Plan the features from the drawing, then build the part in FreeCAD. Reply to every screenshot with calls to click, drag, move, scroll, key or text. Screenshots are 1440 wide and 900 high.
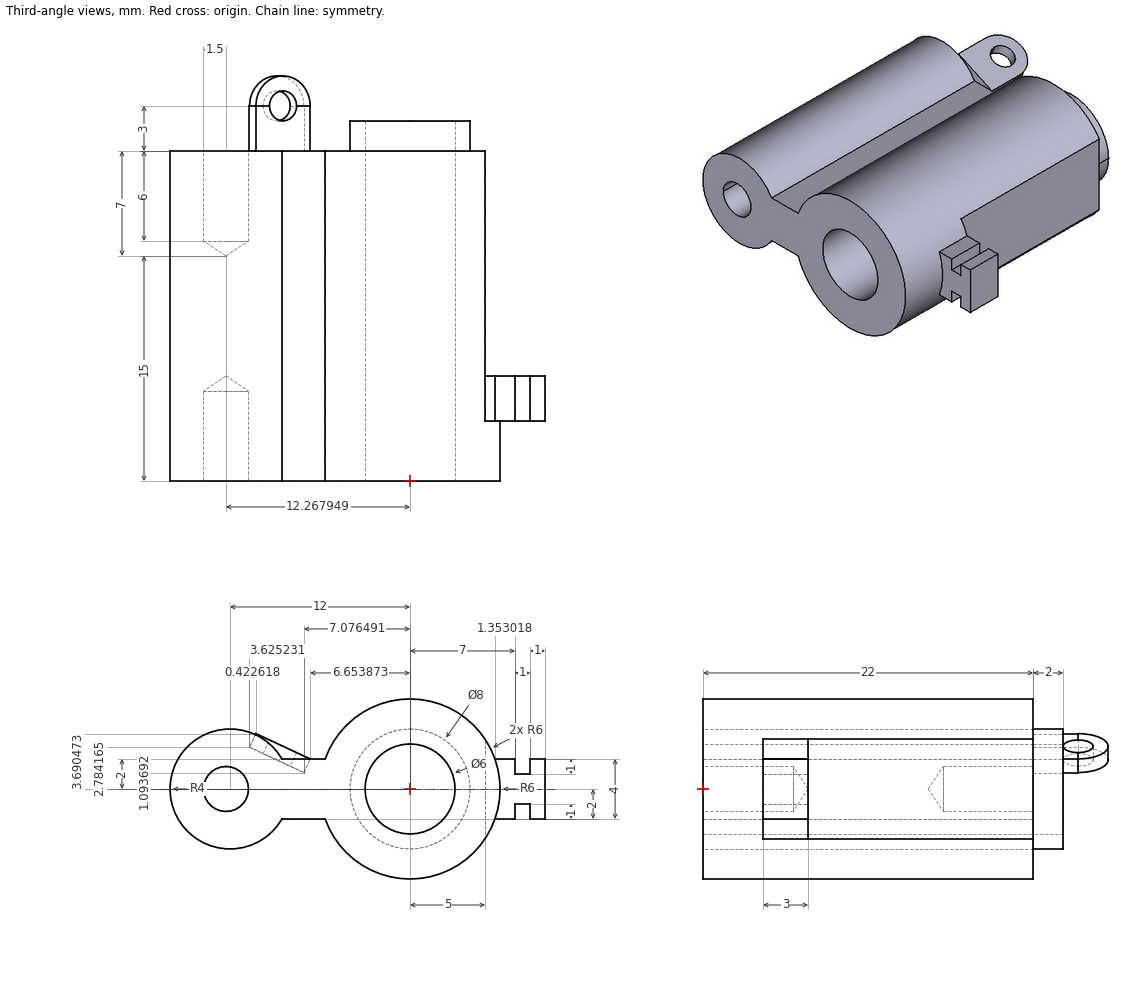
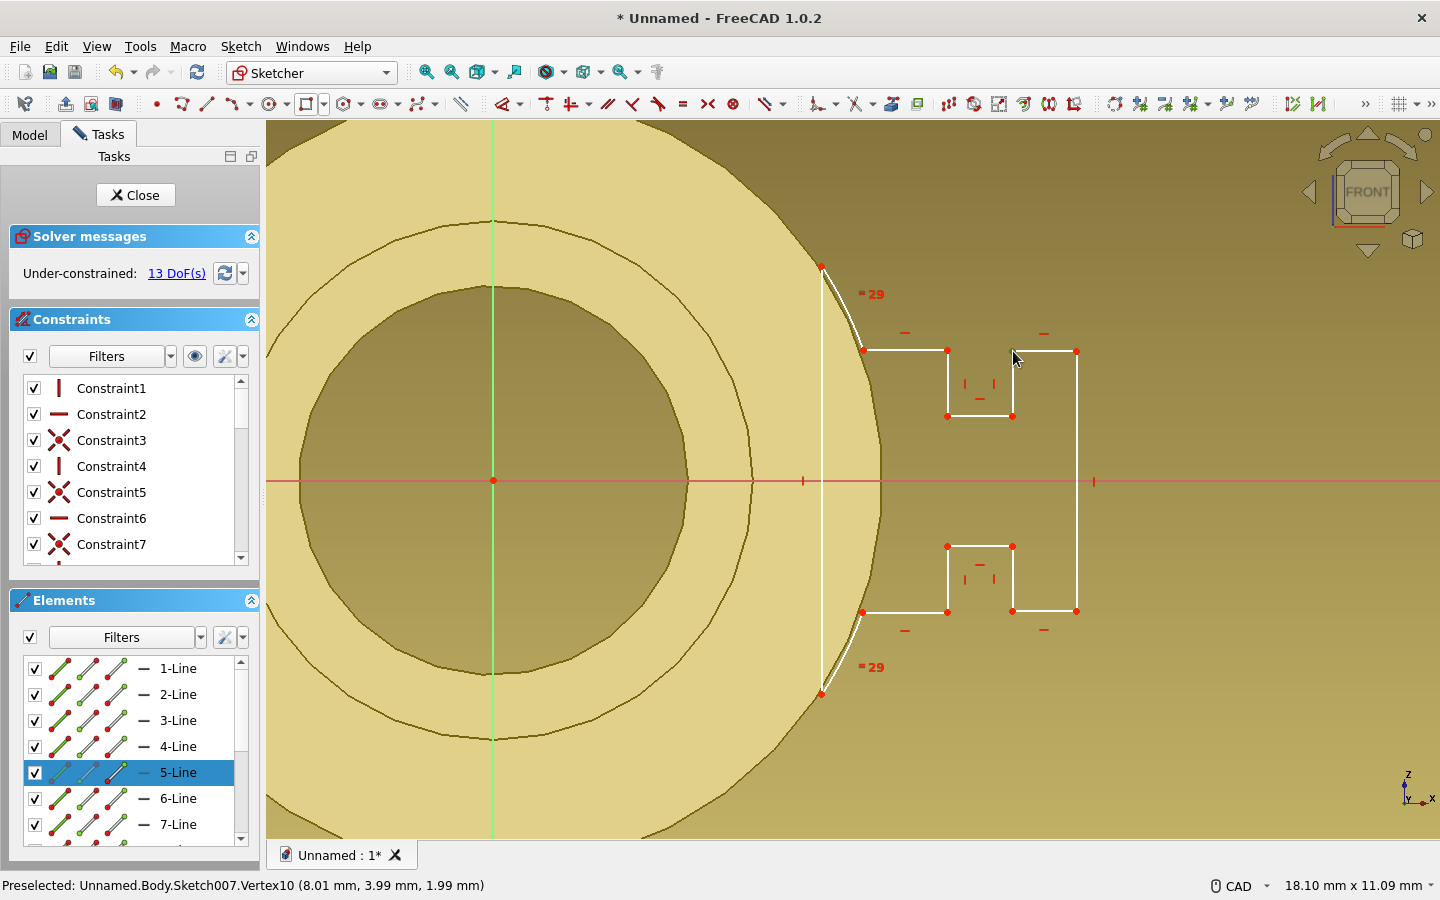
click(1013, 611)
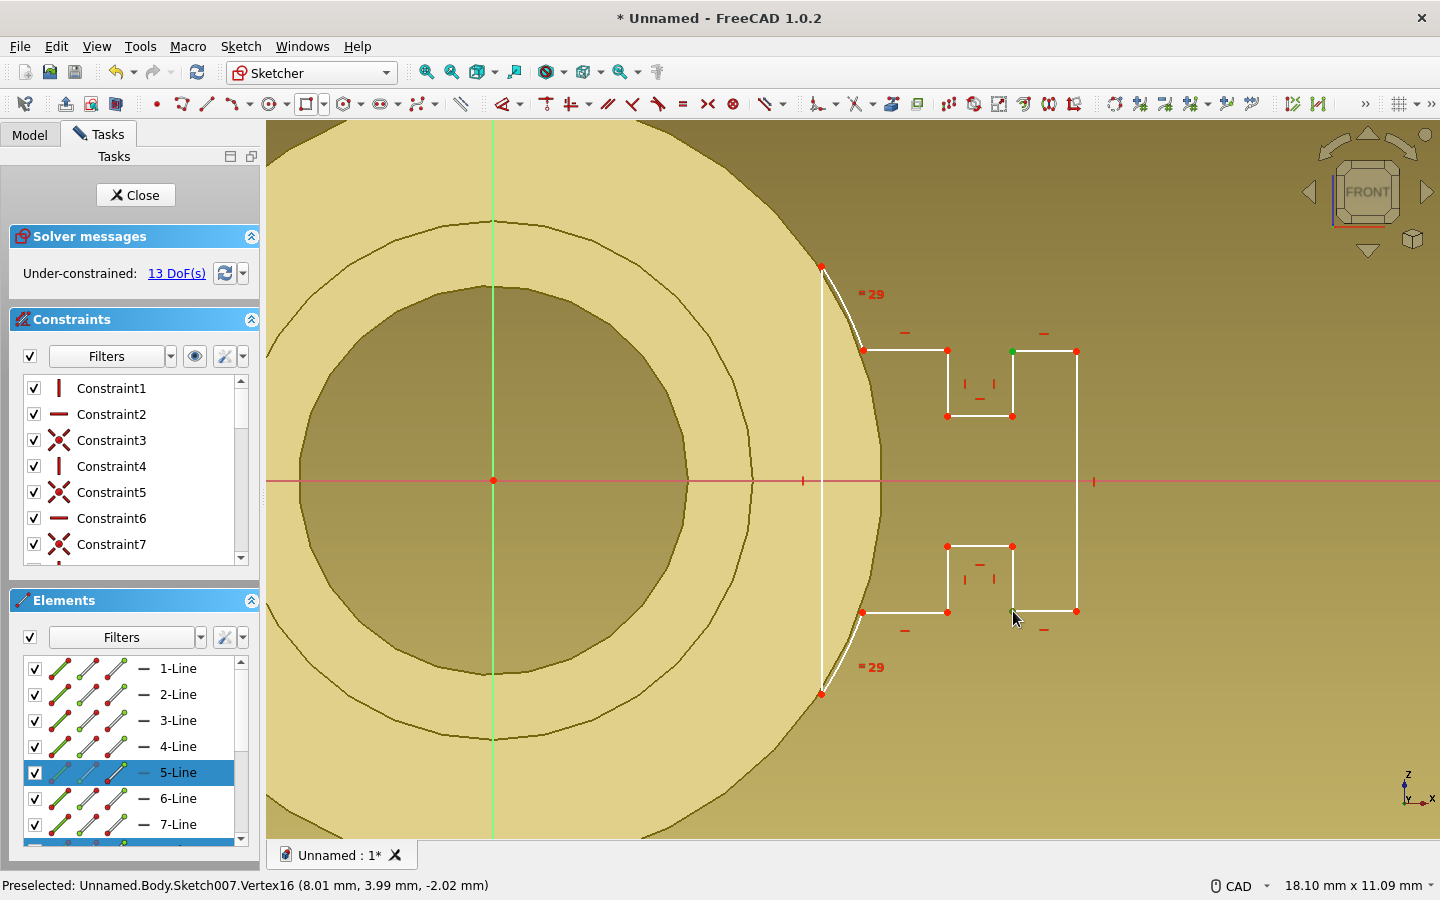
click(364, 481)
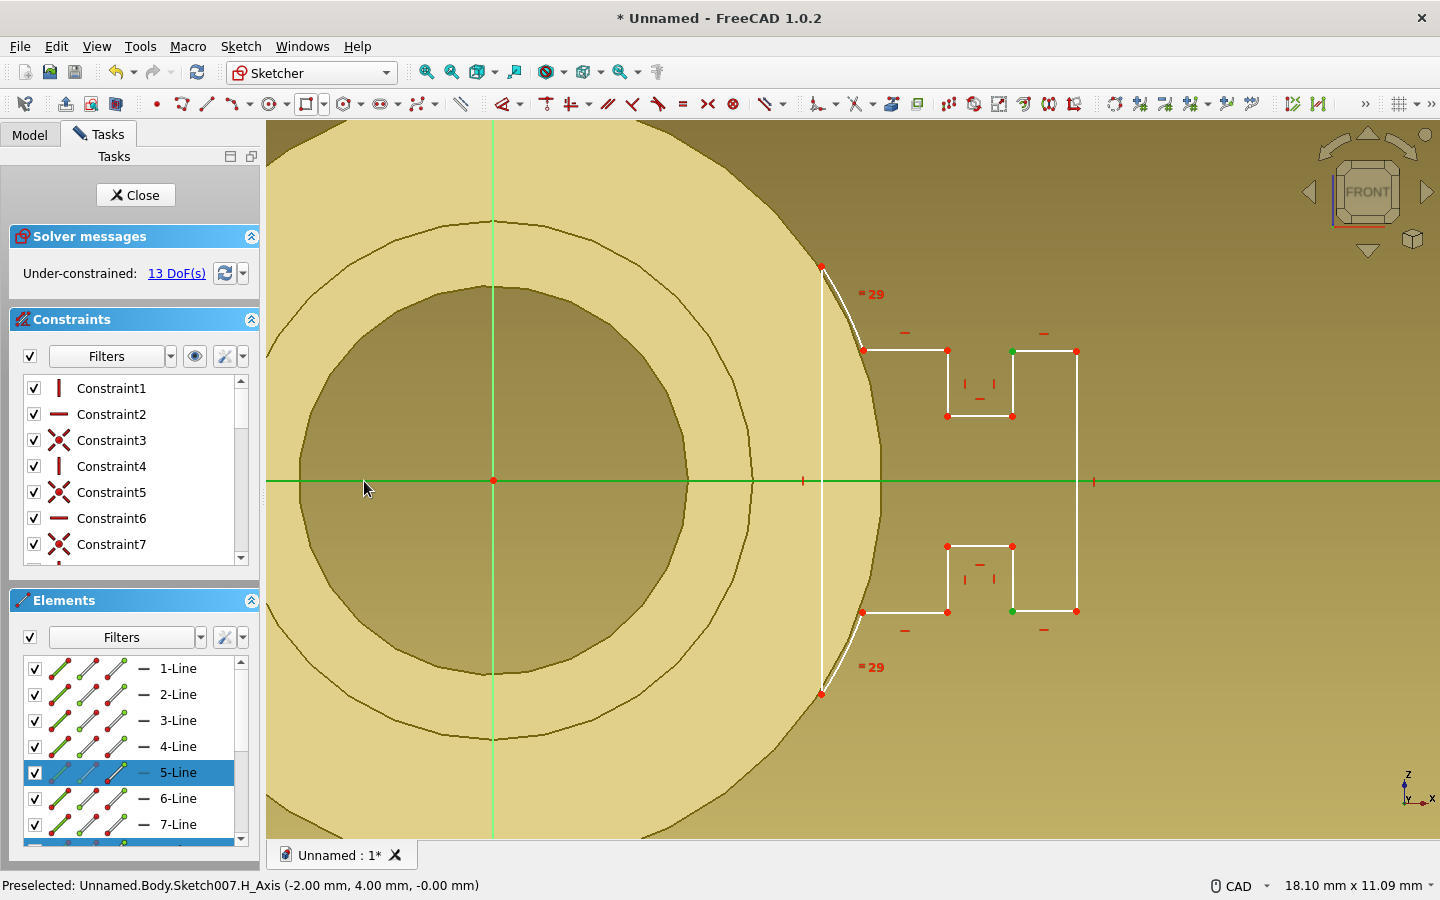
click(708, 104)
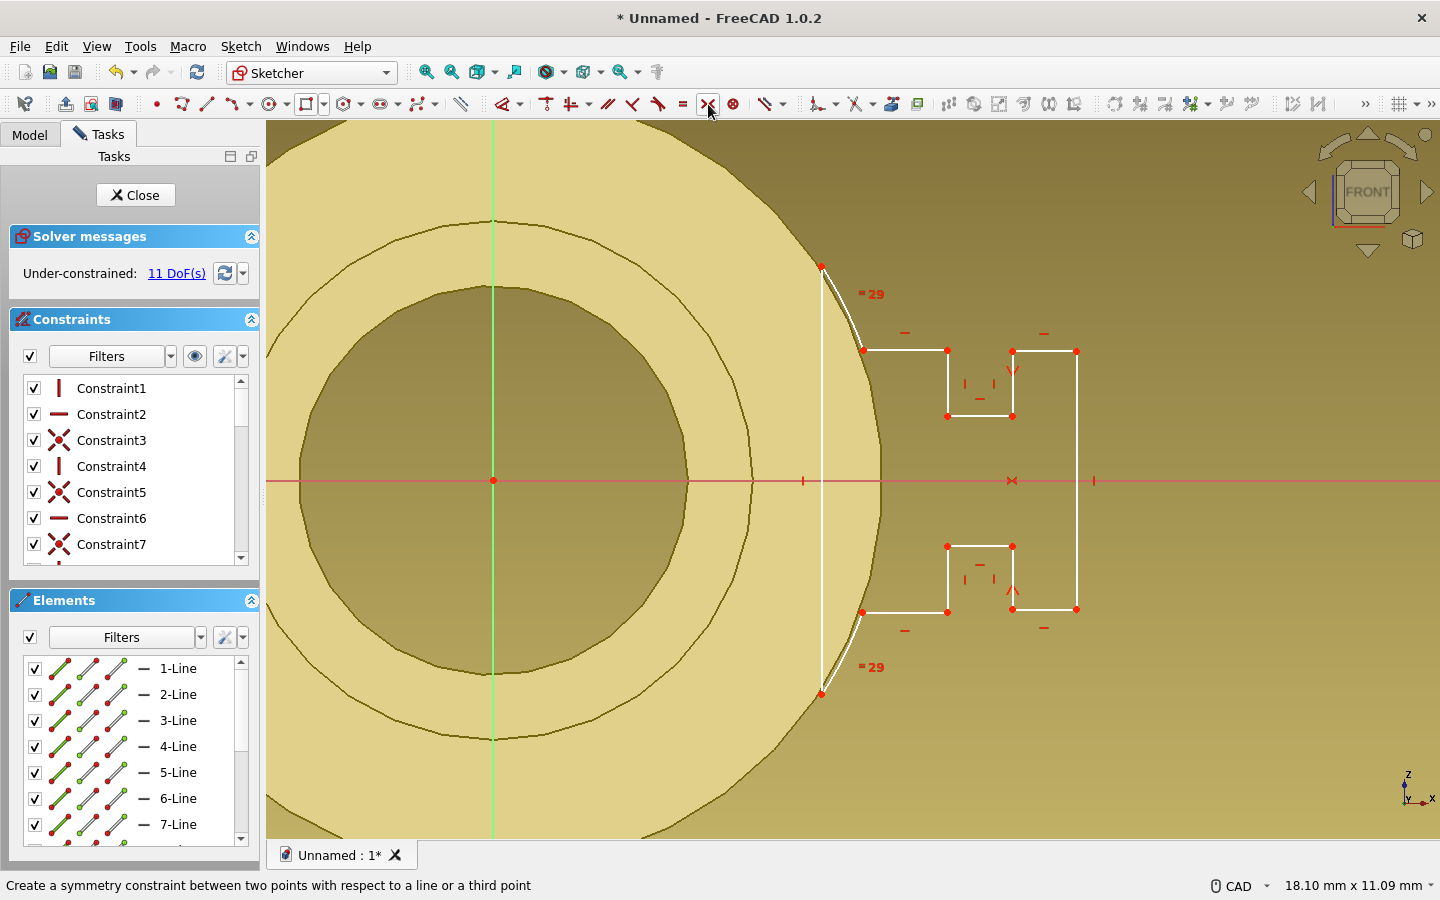
click(948, 416)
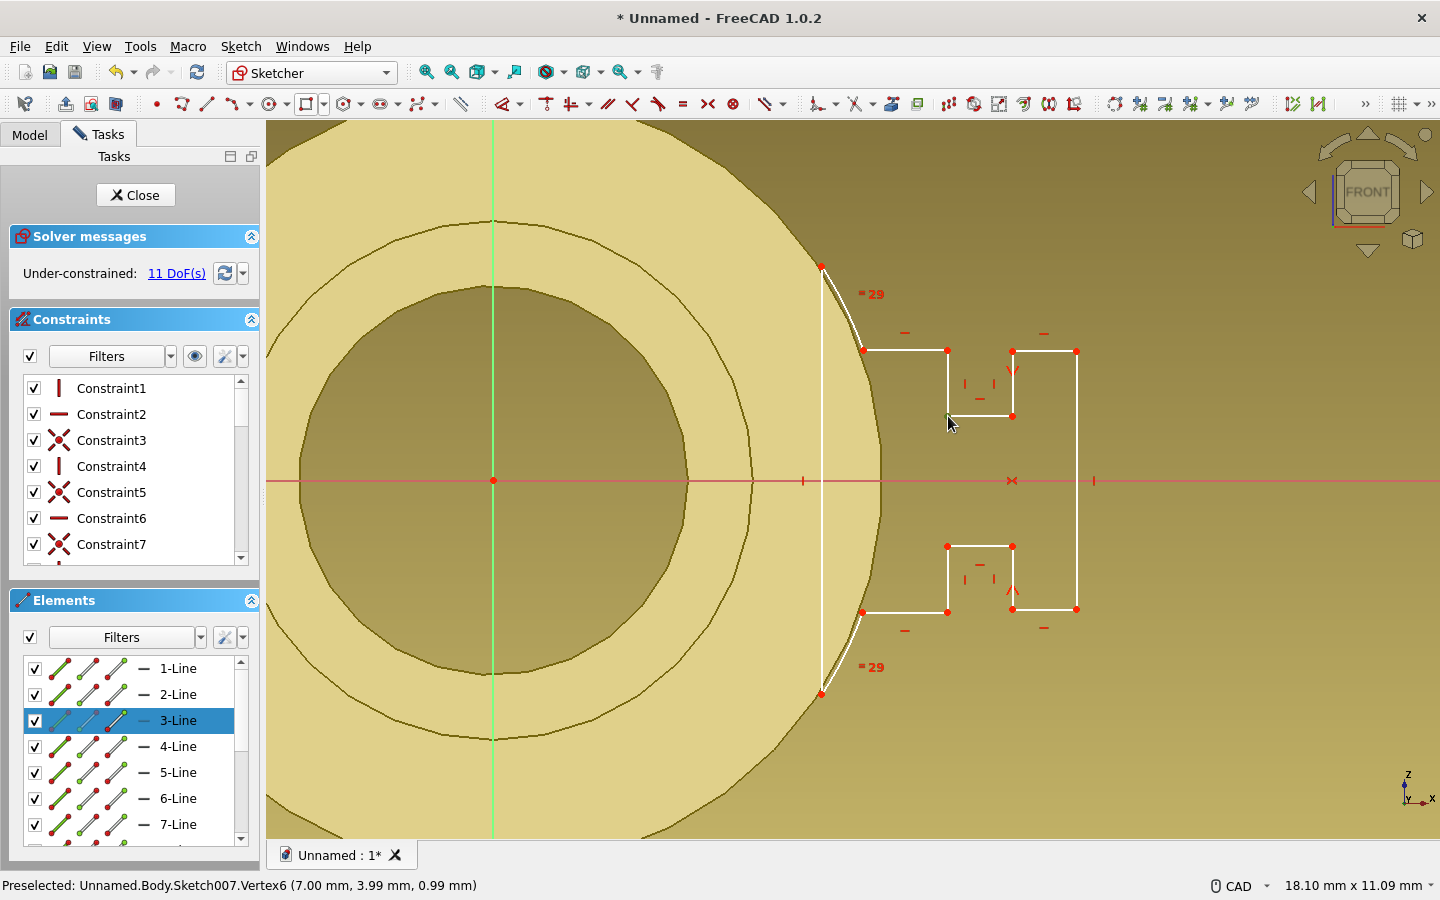
click(948, 546)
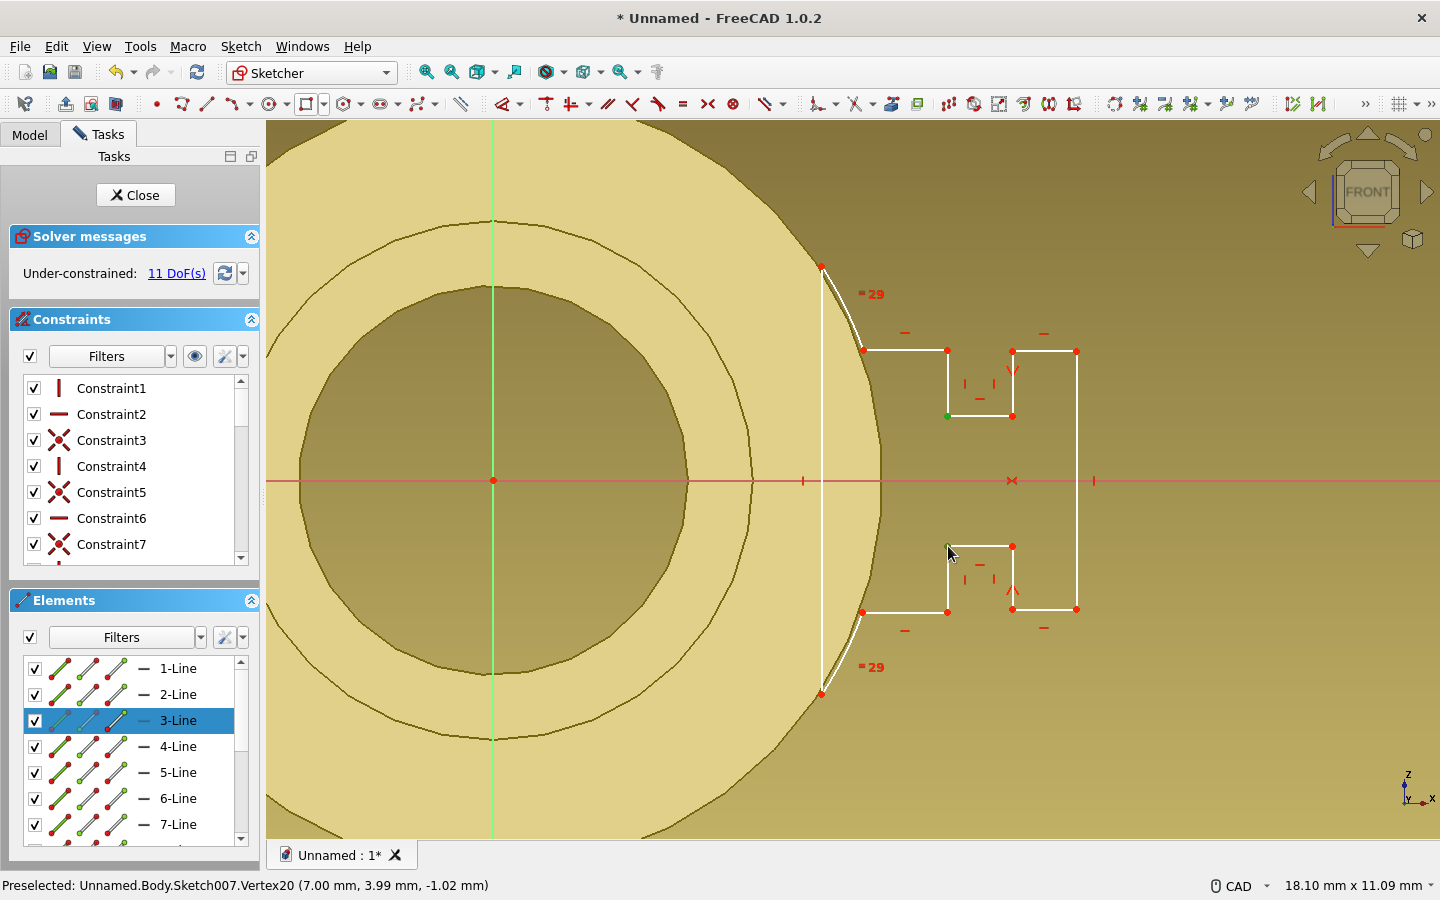
click(364, 481)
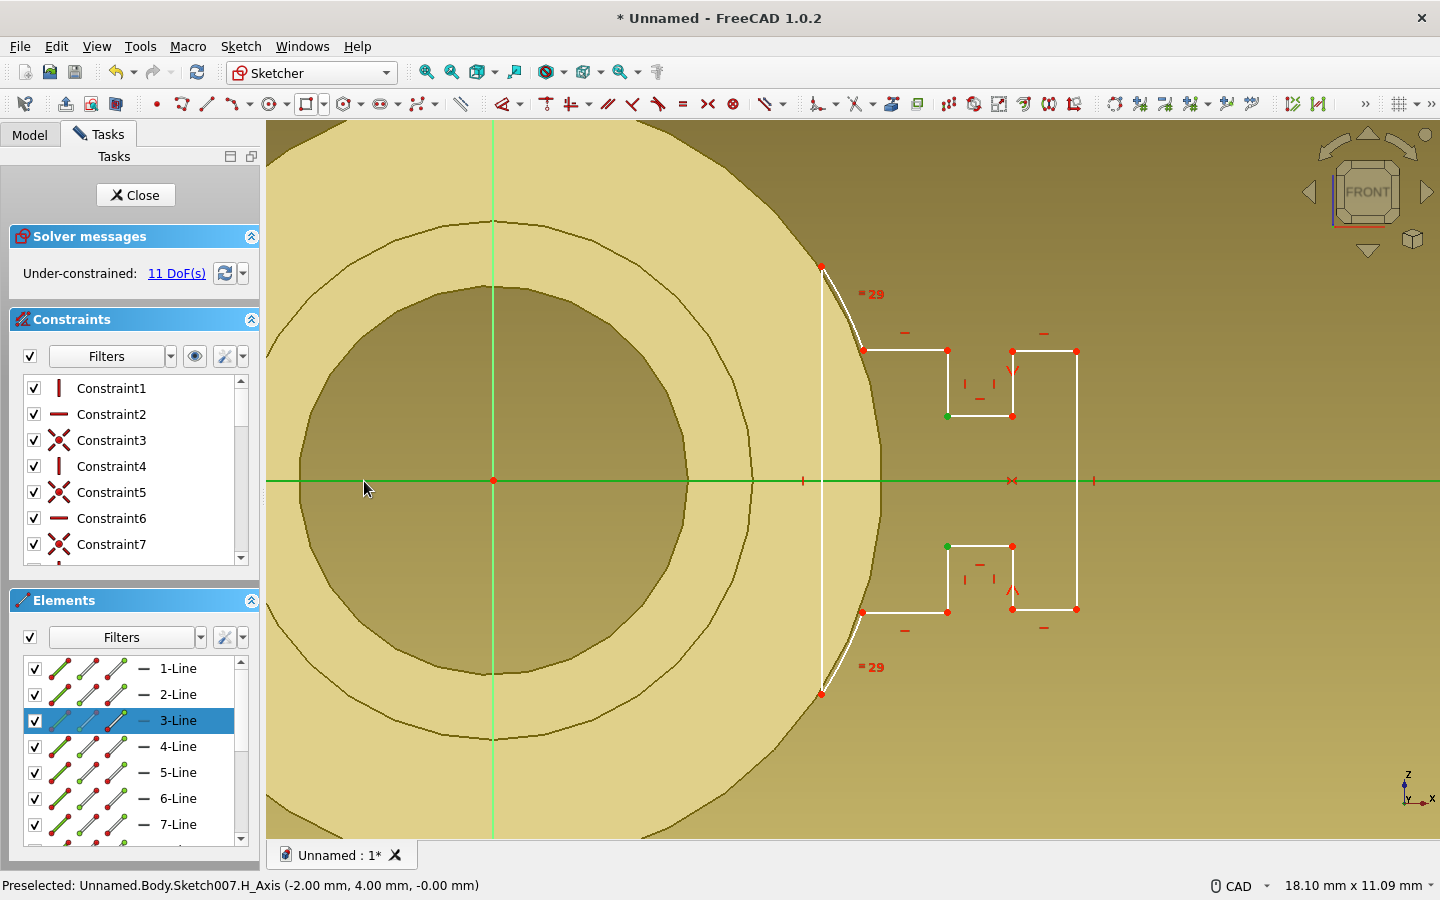
click(708, 104)